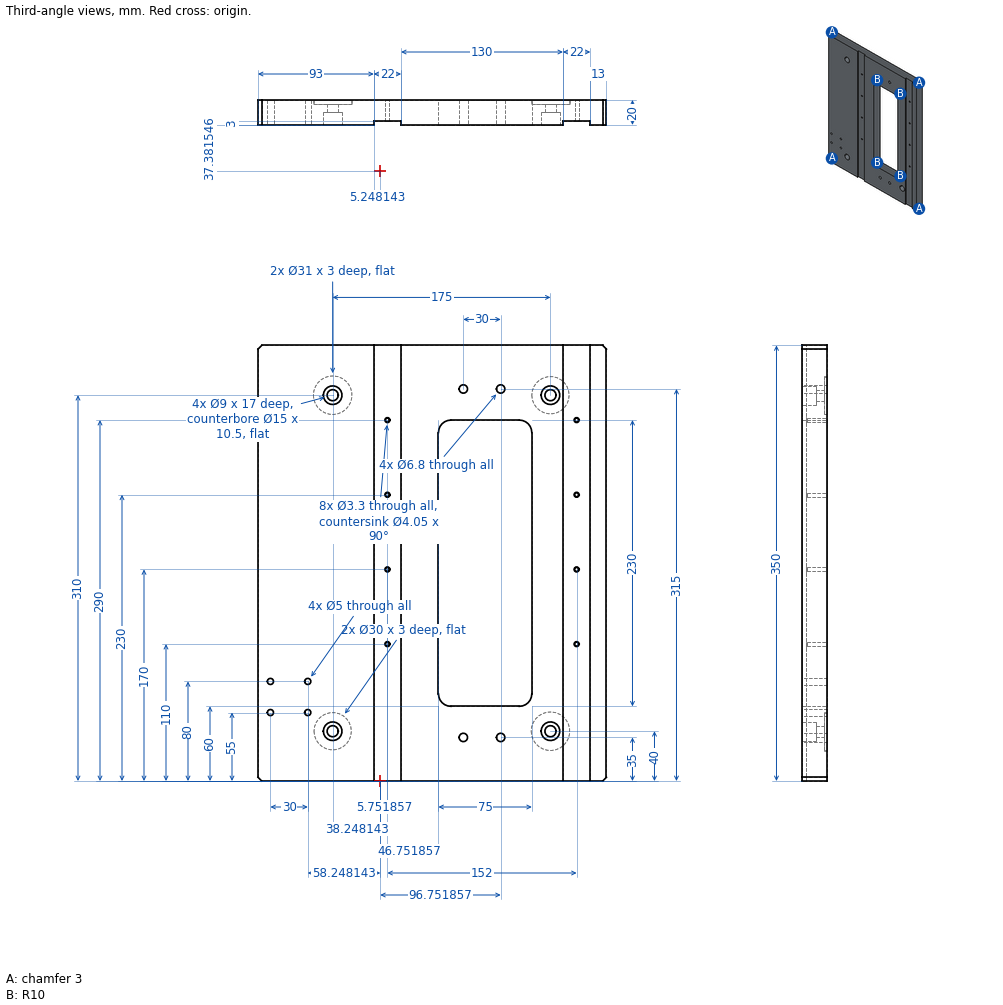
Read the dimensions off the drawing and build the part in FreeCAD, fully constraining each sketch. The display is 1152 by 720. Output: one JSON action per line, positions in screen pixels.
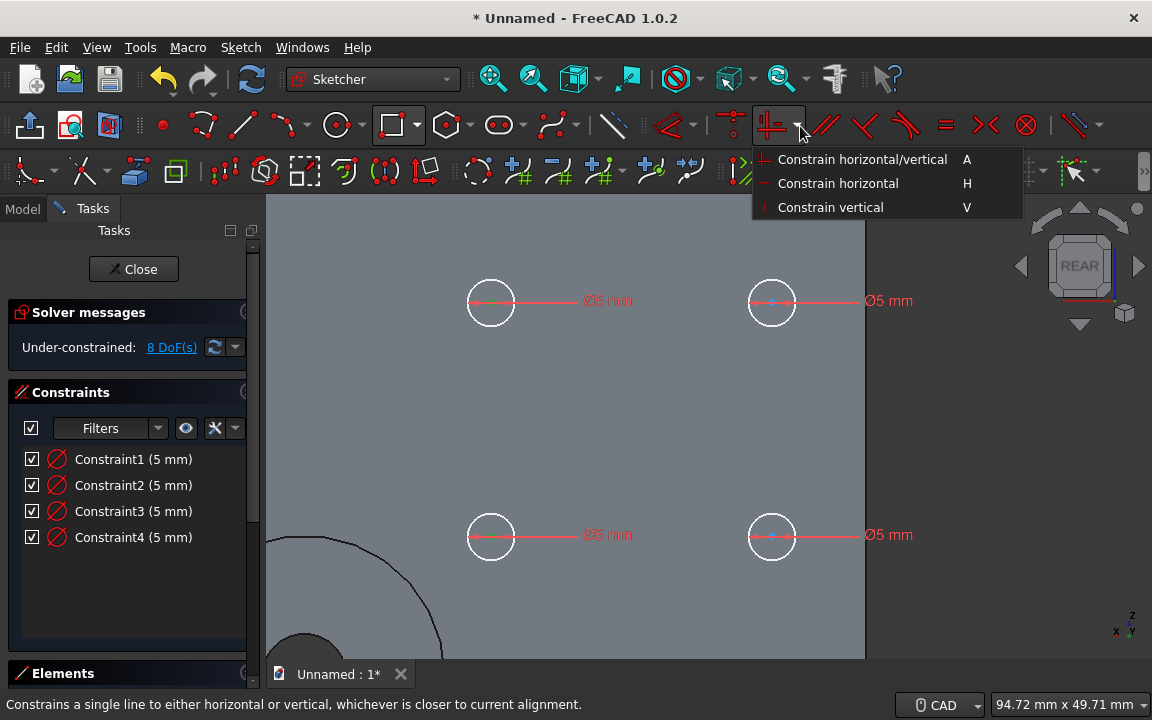
{"action": "left_click", "coordinate": [888, 207]}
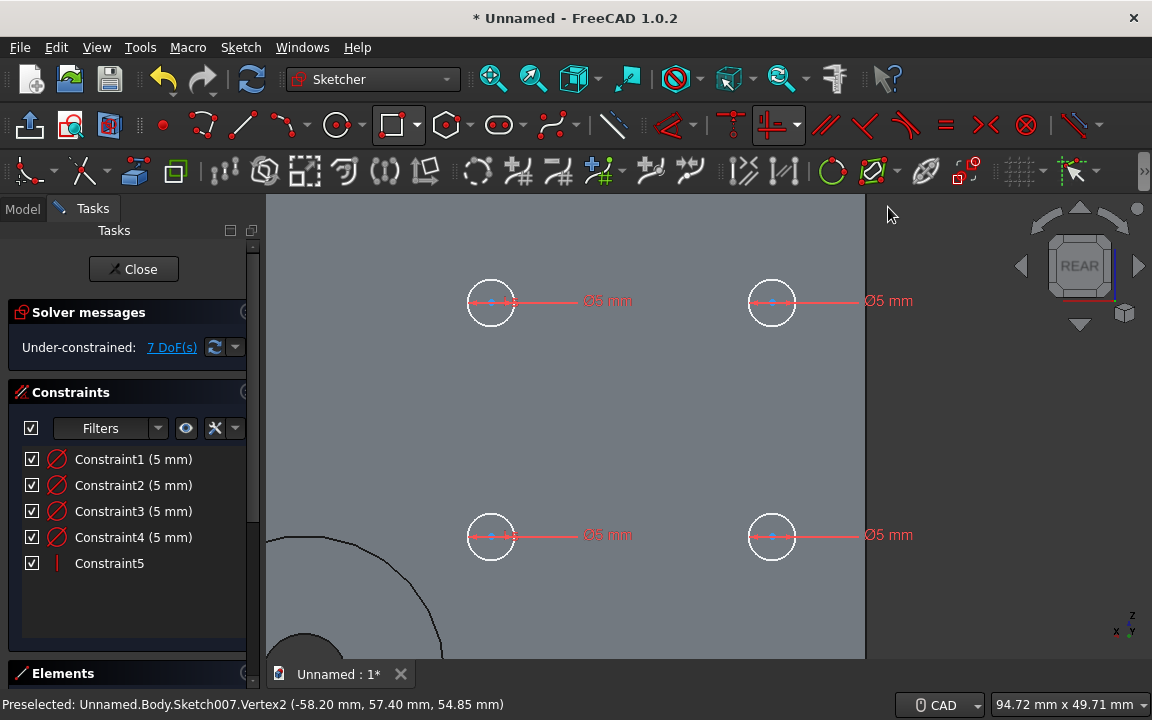
{"action": "left_click", "coordinate": [491, 537]}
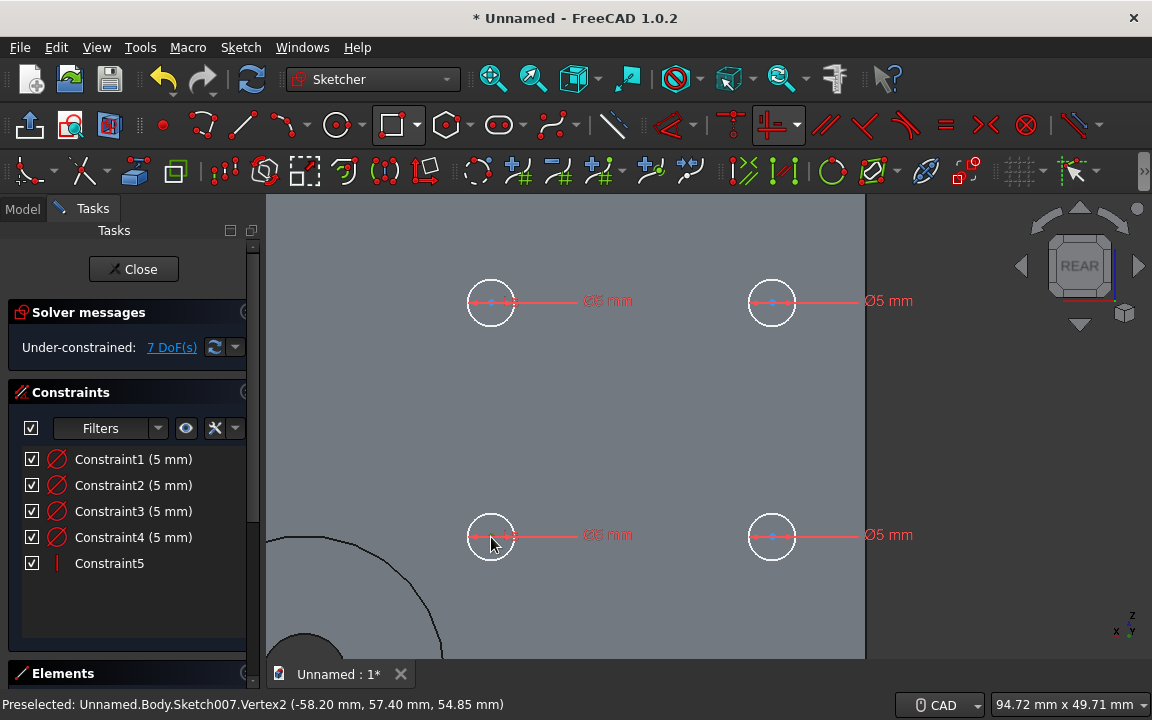
{"action": "left_click", "coordinate": [772, 537]}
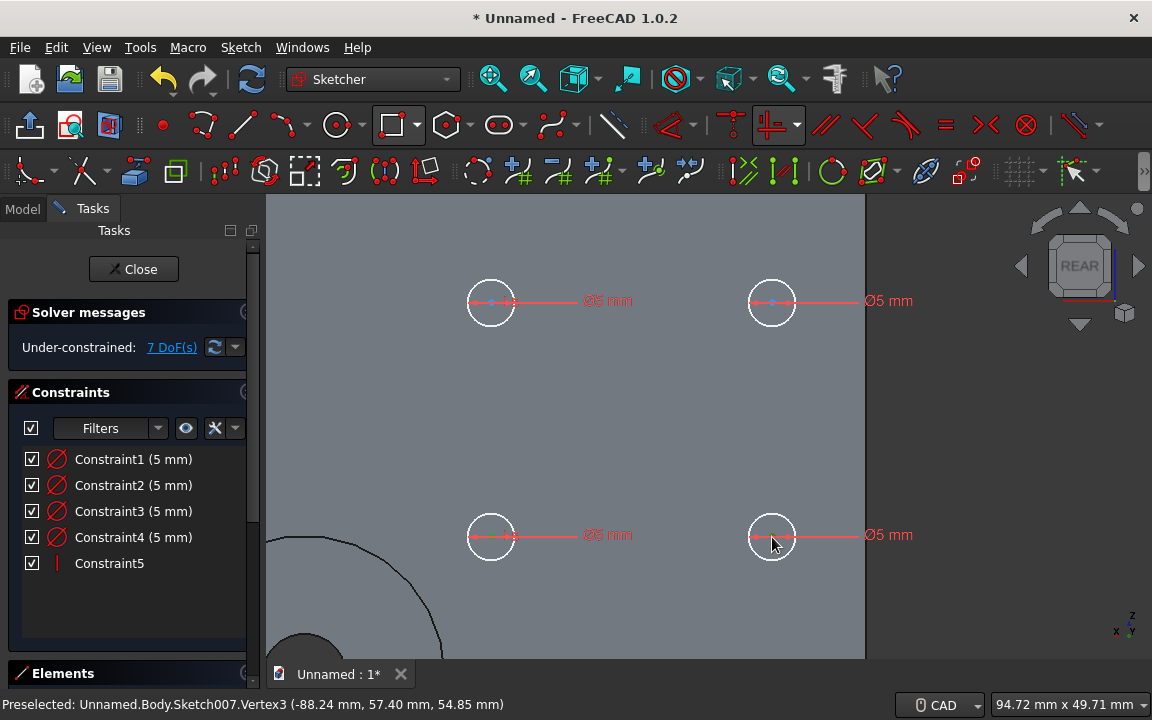
{"action": "left_click", "coordinate": [800, 126]}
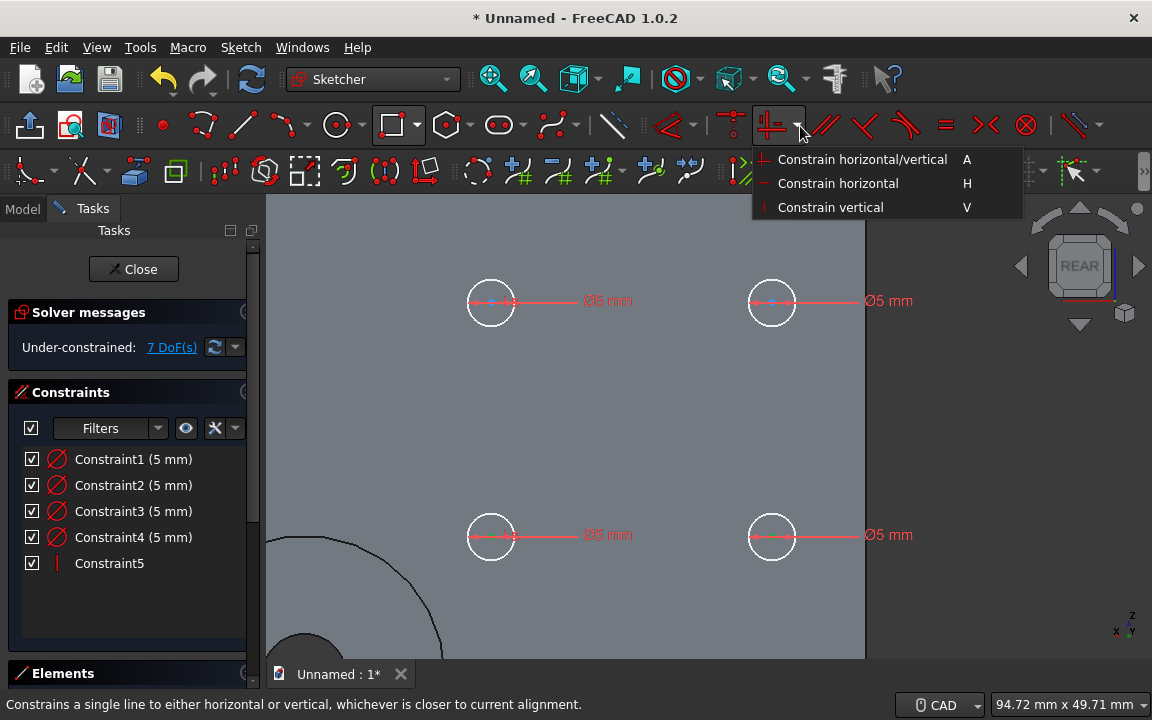
{"action": "left_click", "coordinate": [888, 183]}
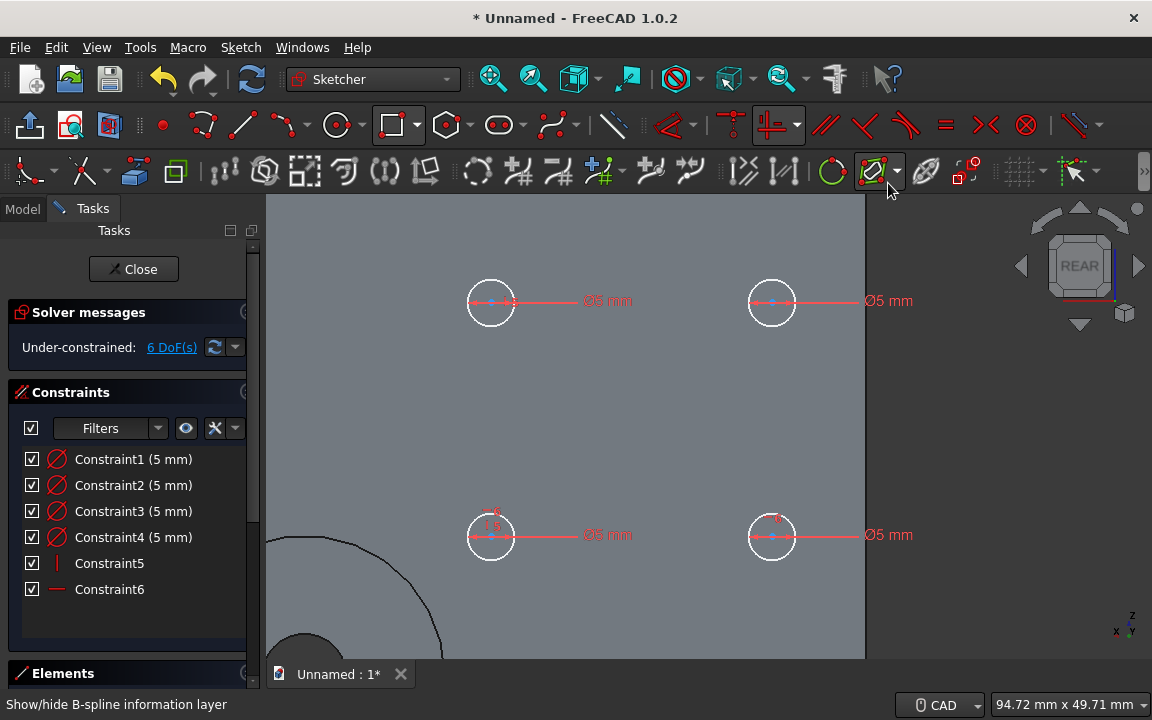
{"action": "left_click", "coordinate": [772, 537]}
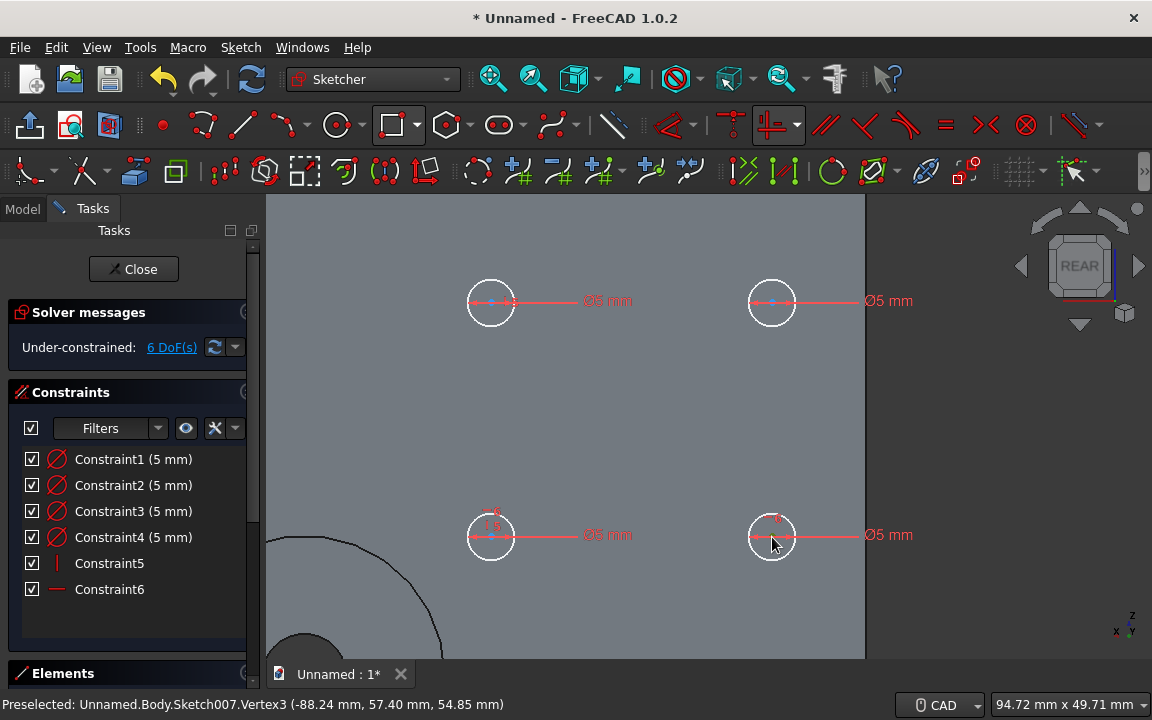
{"action": "left_click", "coordinate": [772, 303]}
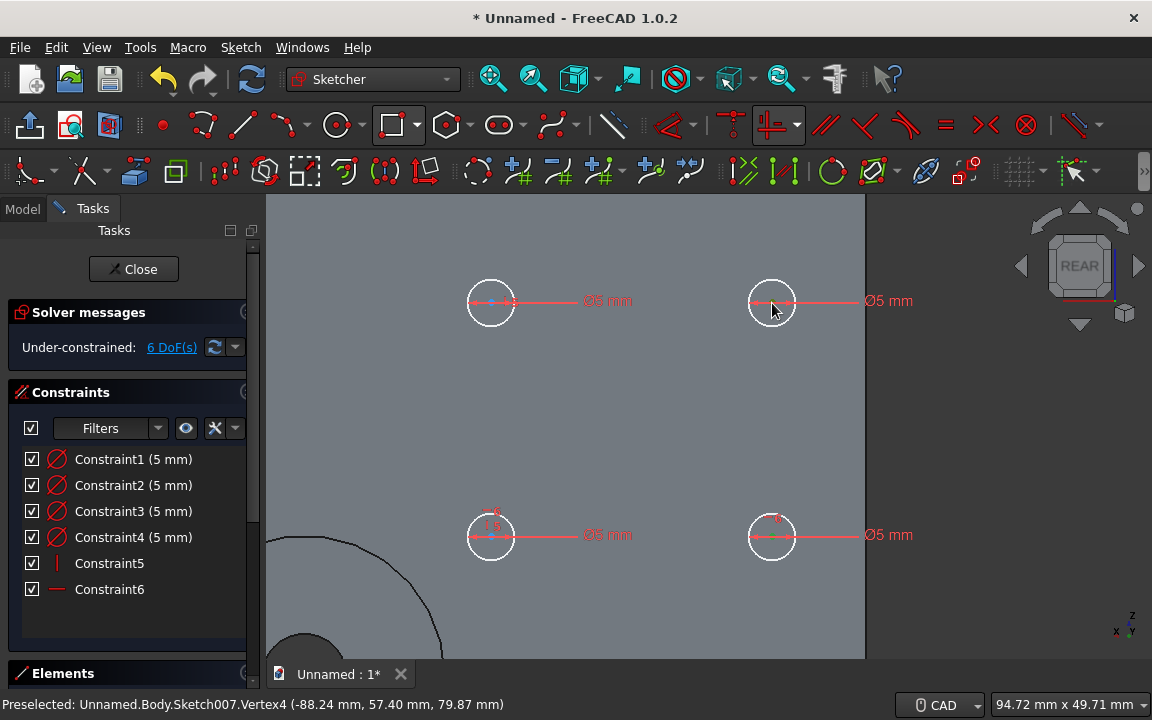
{"action": "left_click", "coordinate": [800, 126]}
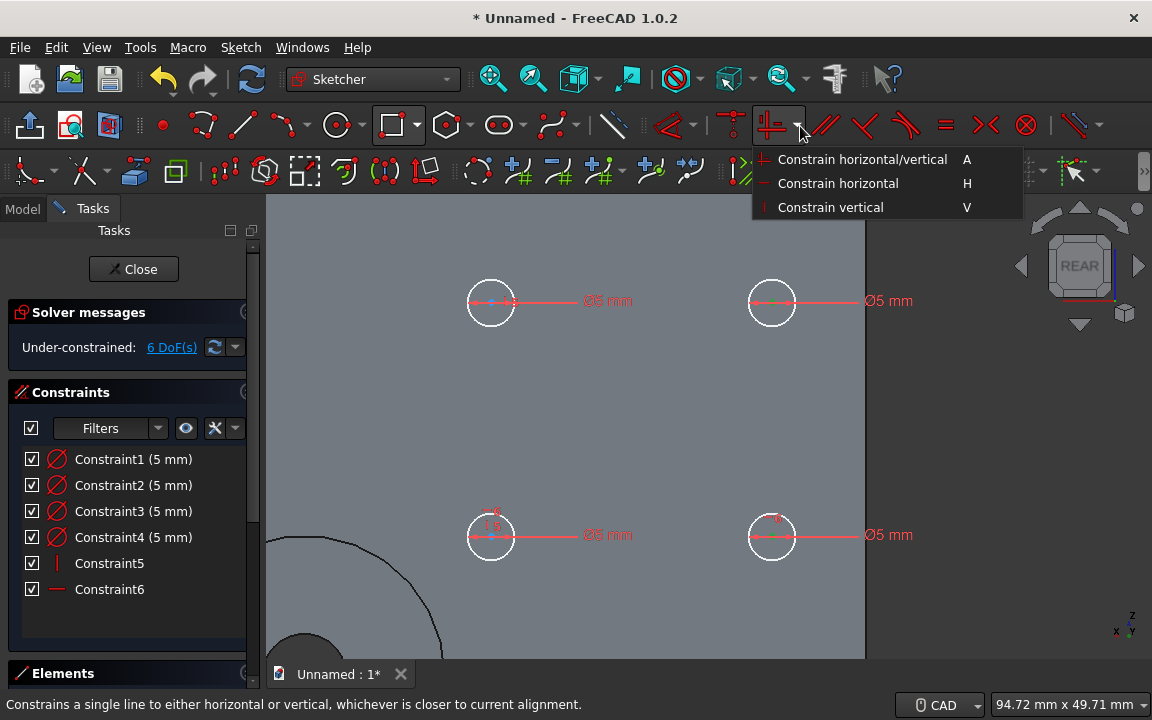
{"action": "left_click", "coordinate": [888, 207]}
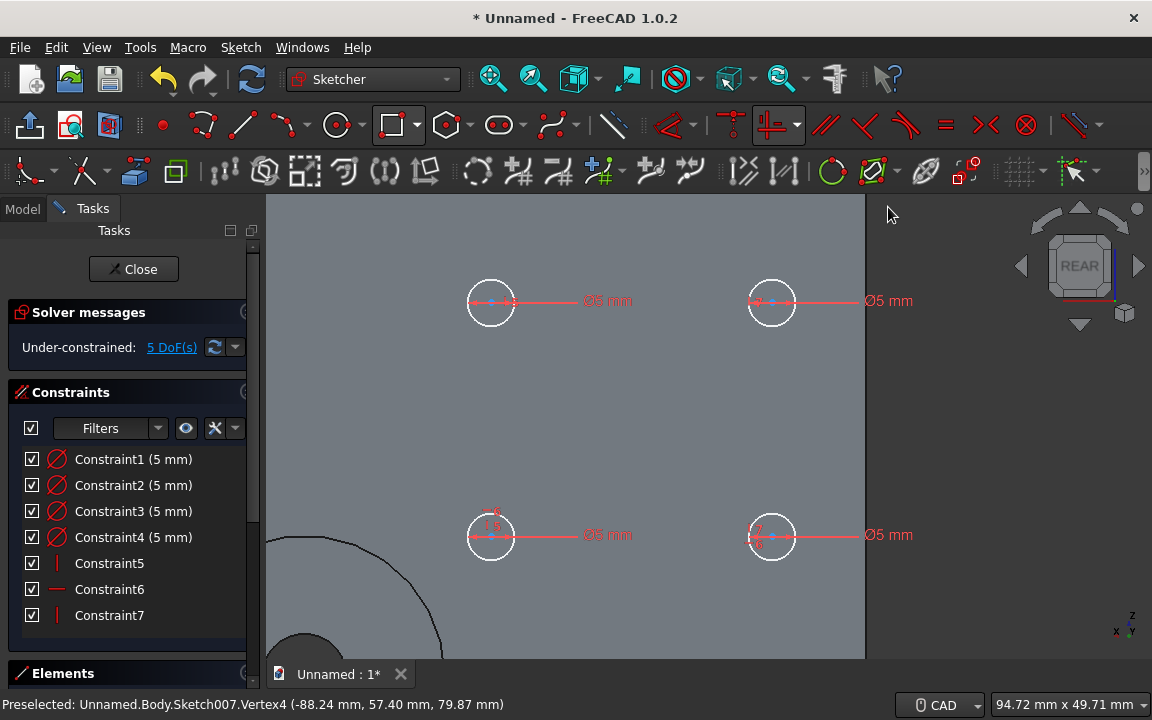
{"action": "left_click", "coordinate": [491, 303]}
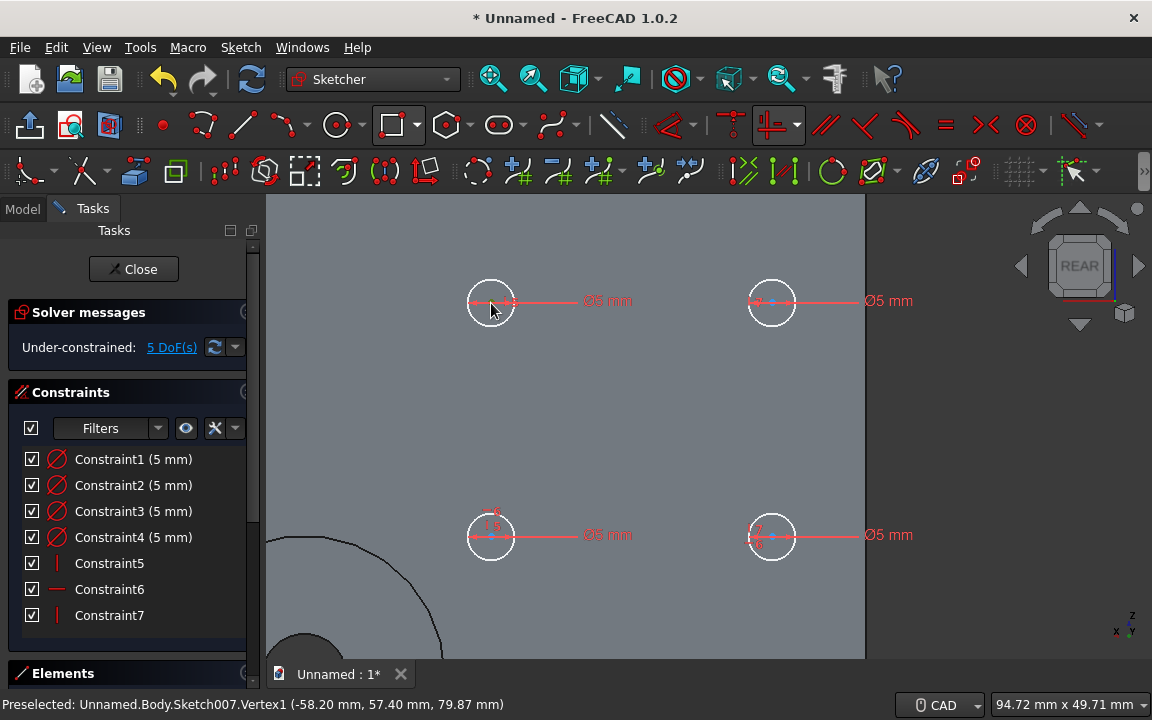
{"action": "left_click", "coordinate": [772, 303]}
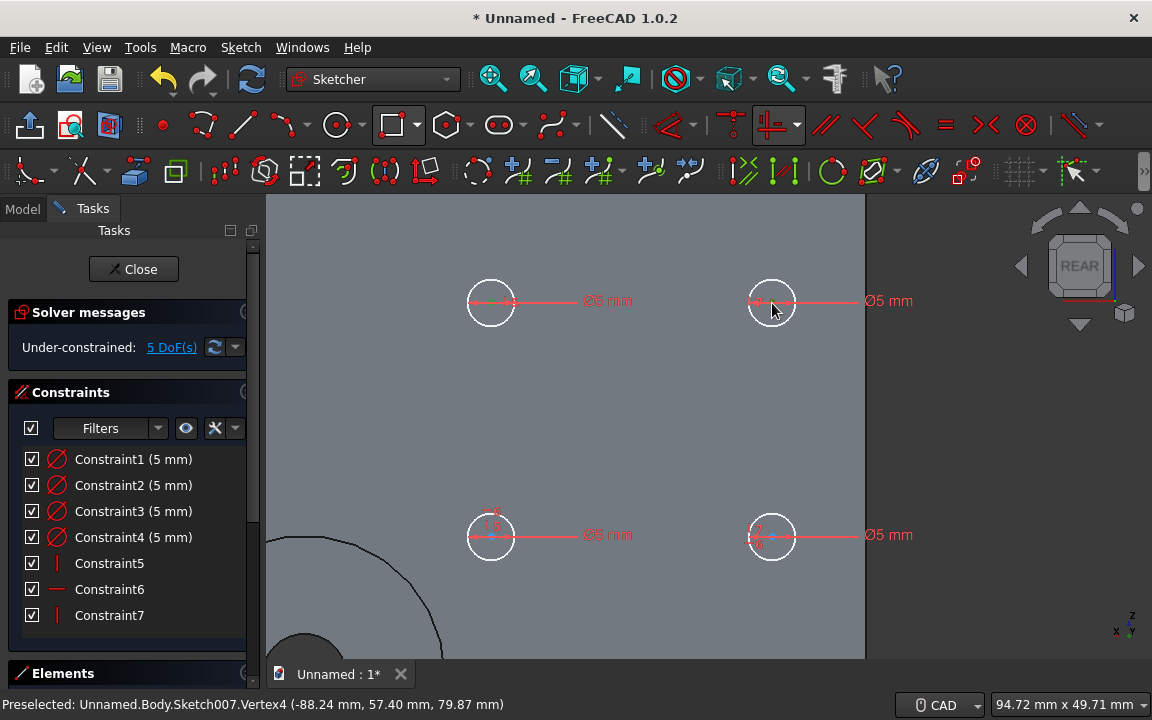
{"action": "left_click", "coordinate": [800, 126]}